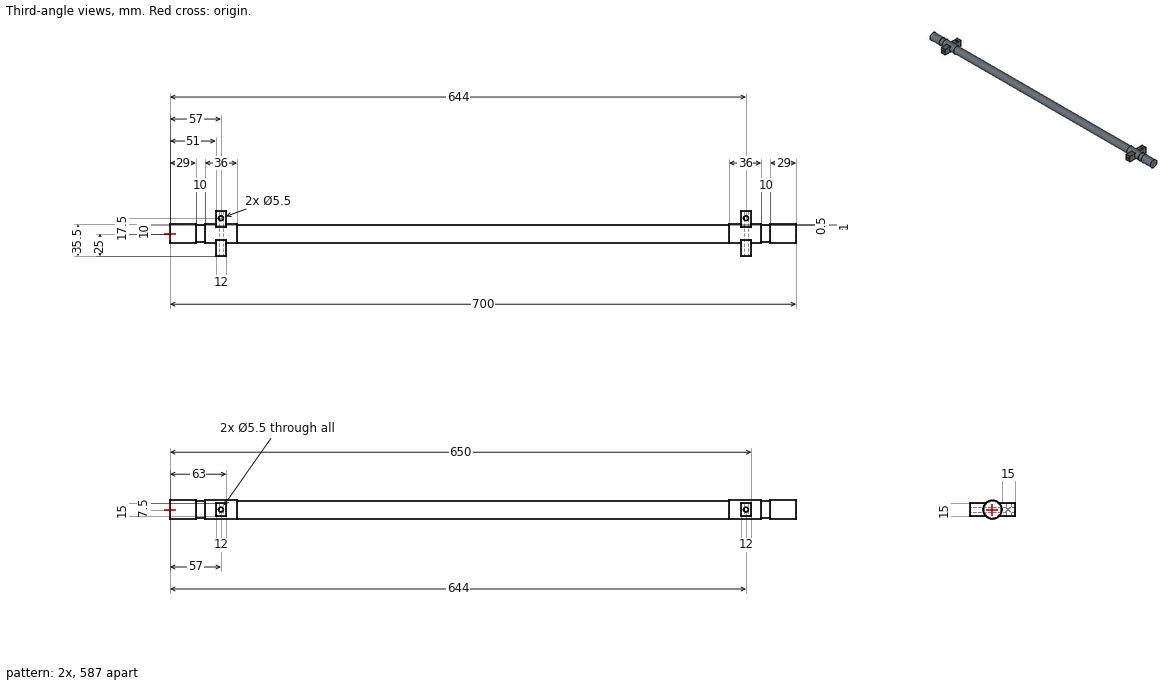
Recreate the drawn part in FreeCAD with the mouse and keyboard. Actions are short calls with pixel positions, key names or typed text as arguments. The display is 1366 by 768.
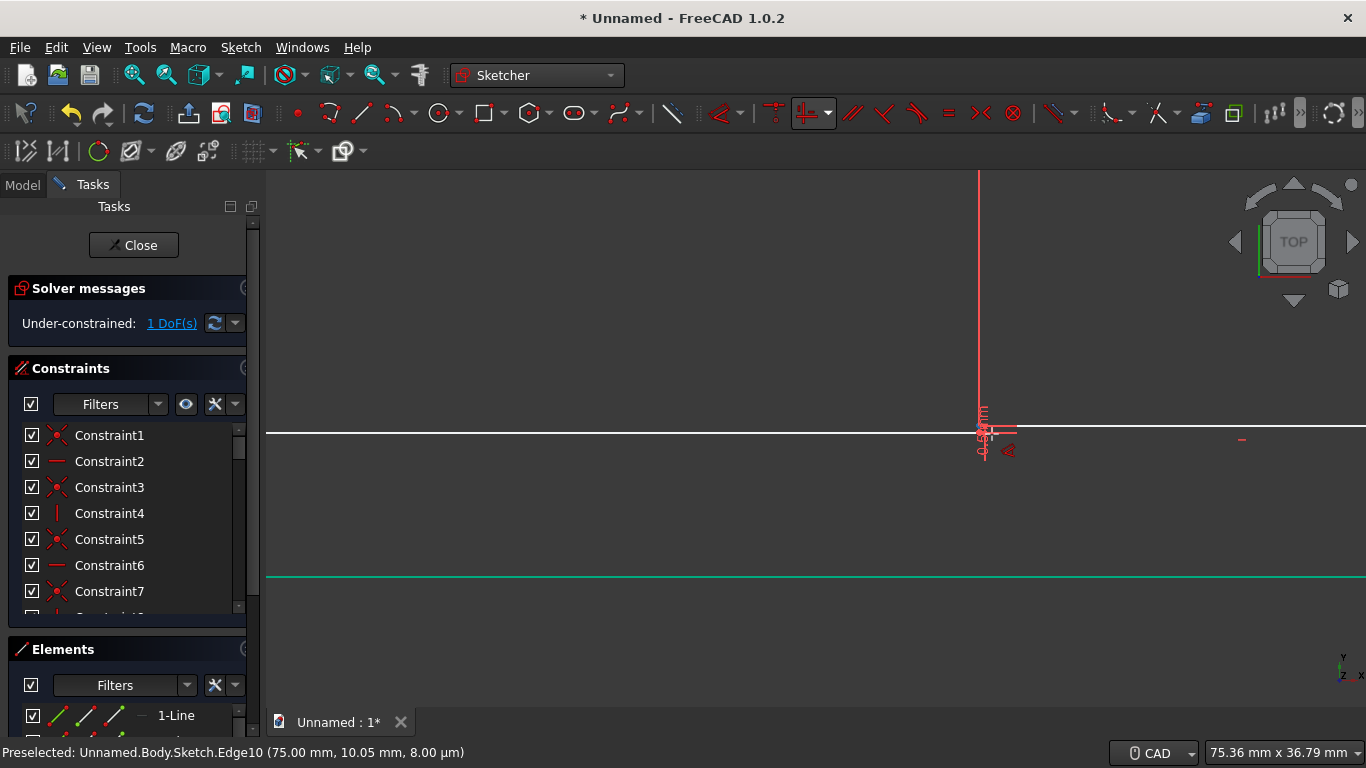
click(979, 433)
click(1013, 505)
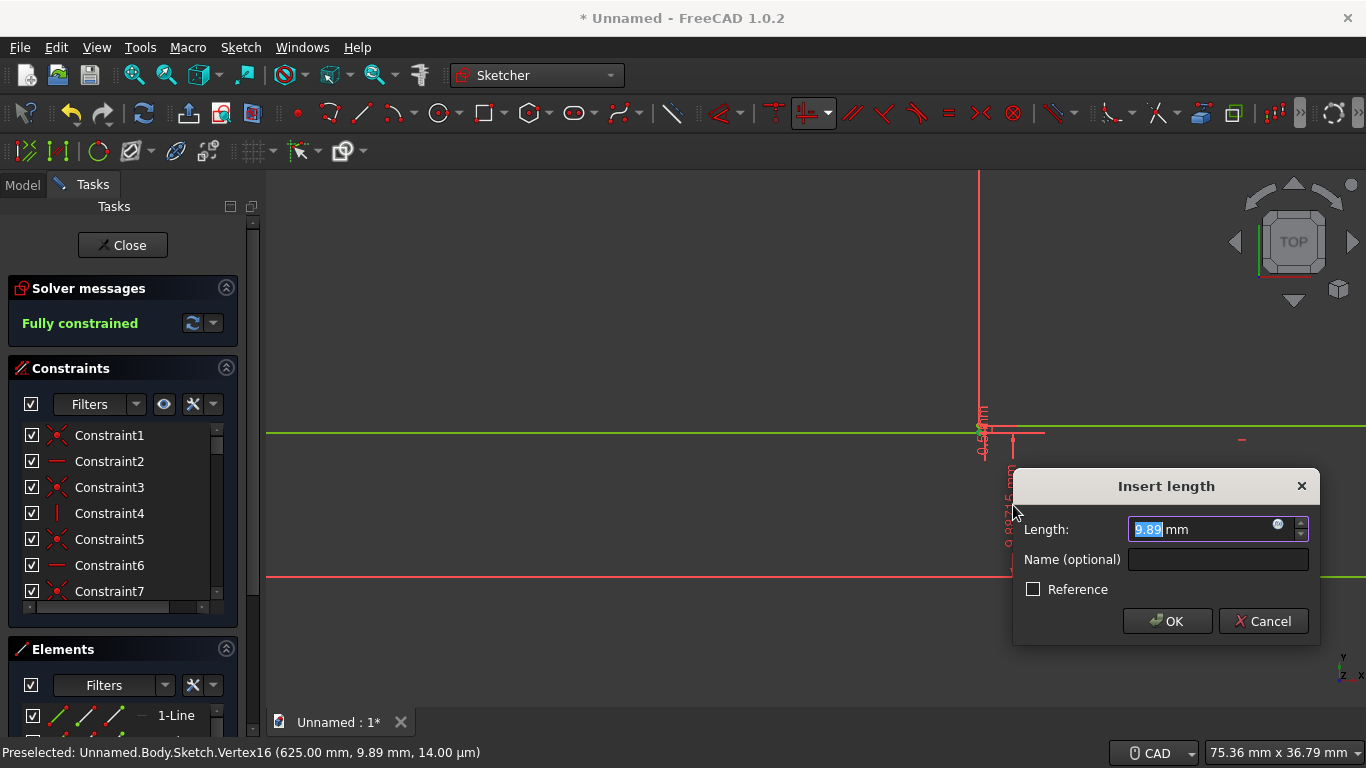
text(10)
key(Return)
key(Escape)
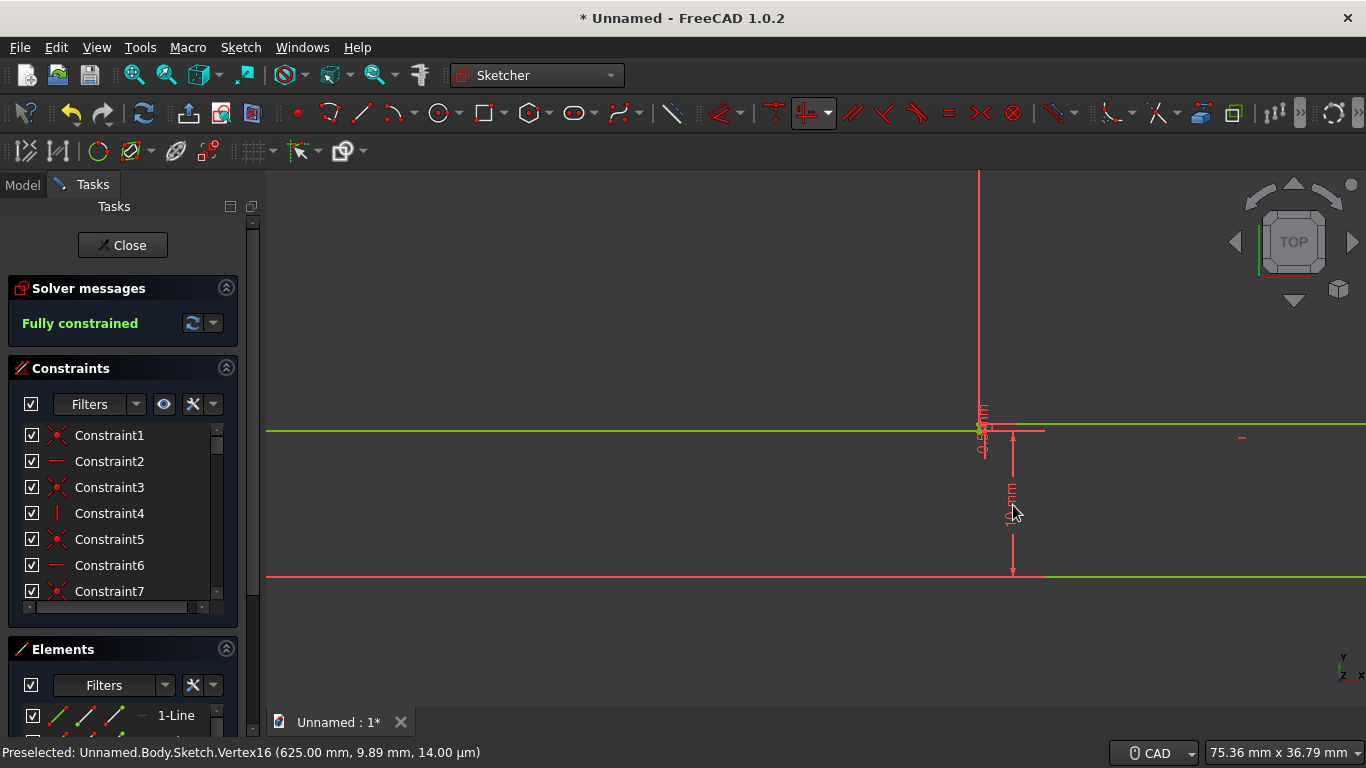
click(123, 245)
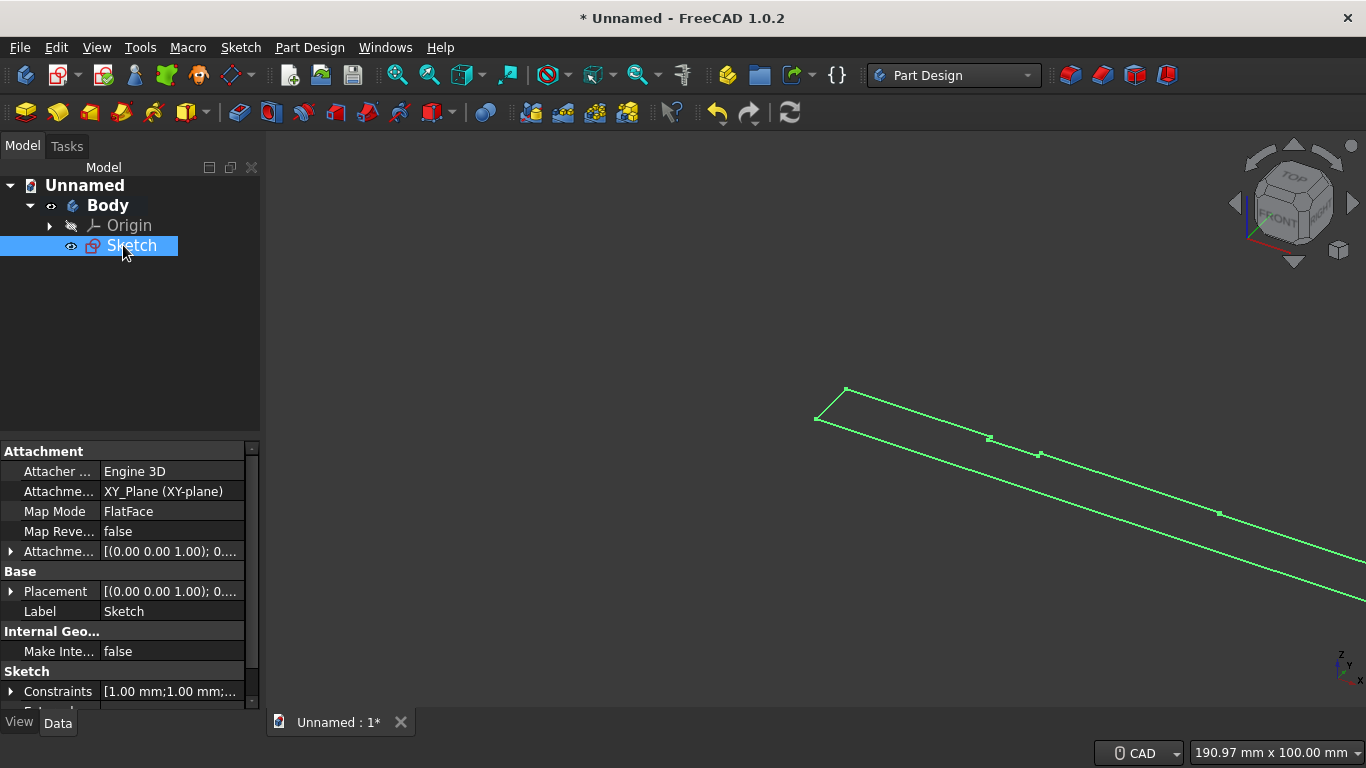
click(58, 112)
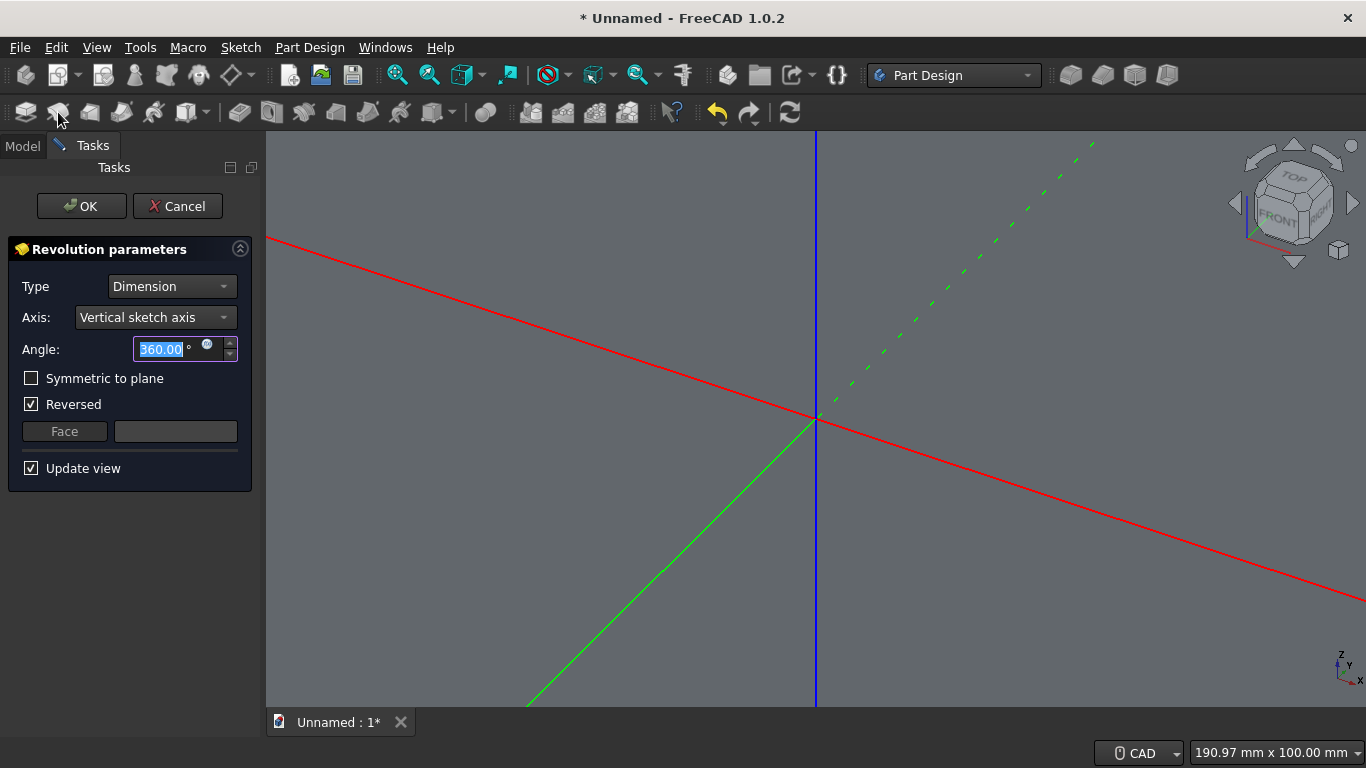
click(156, 318)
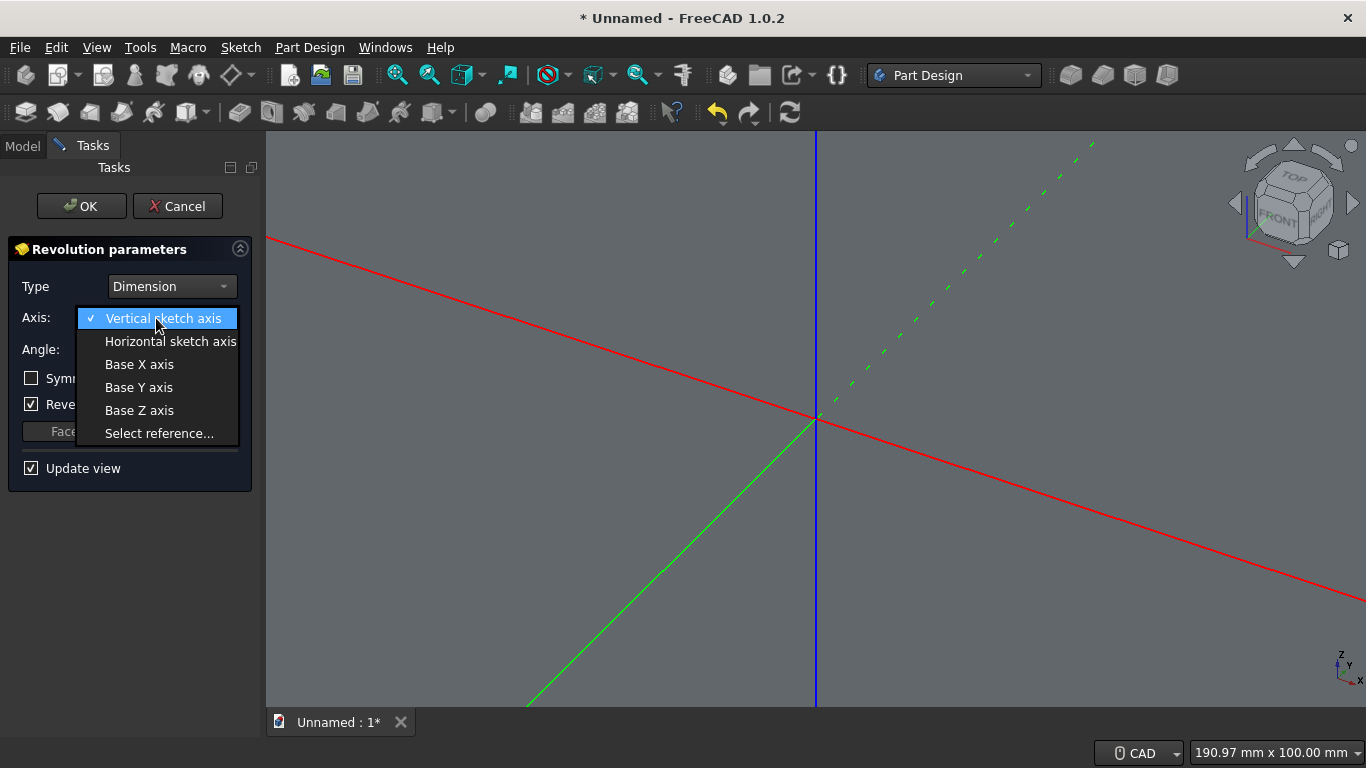
click(156, 342)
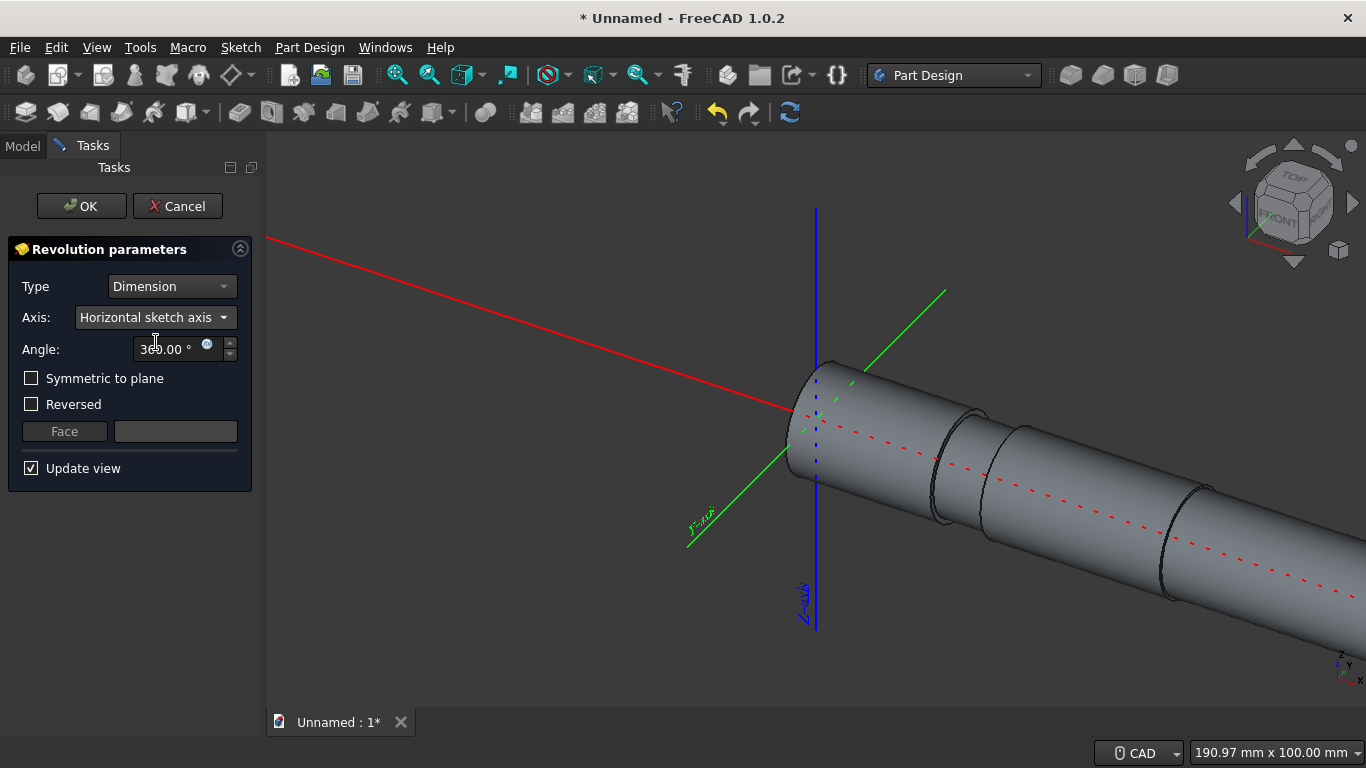
click(82, 206)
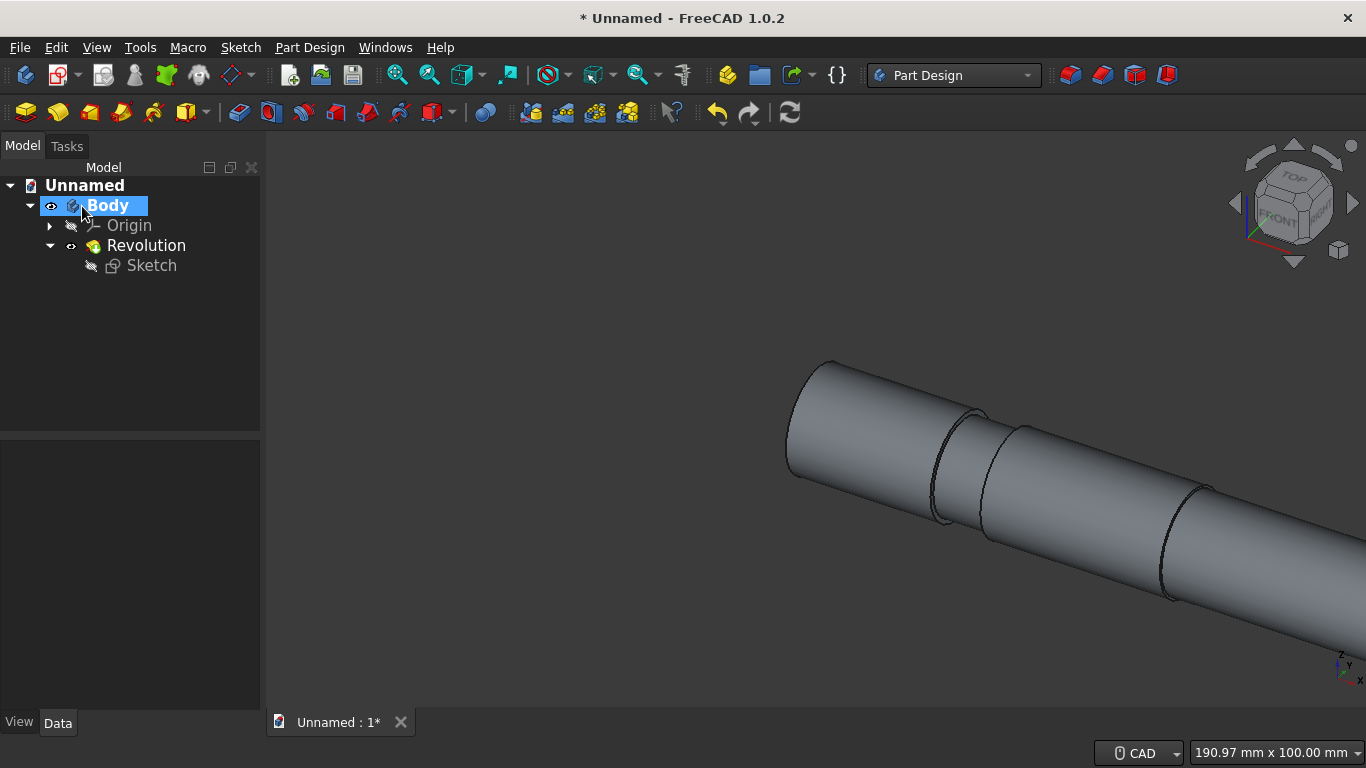
click(398, 76)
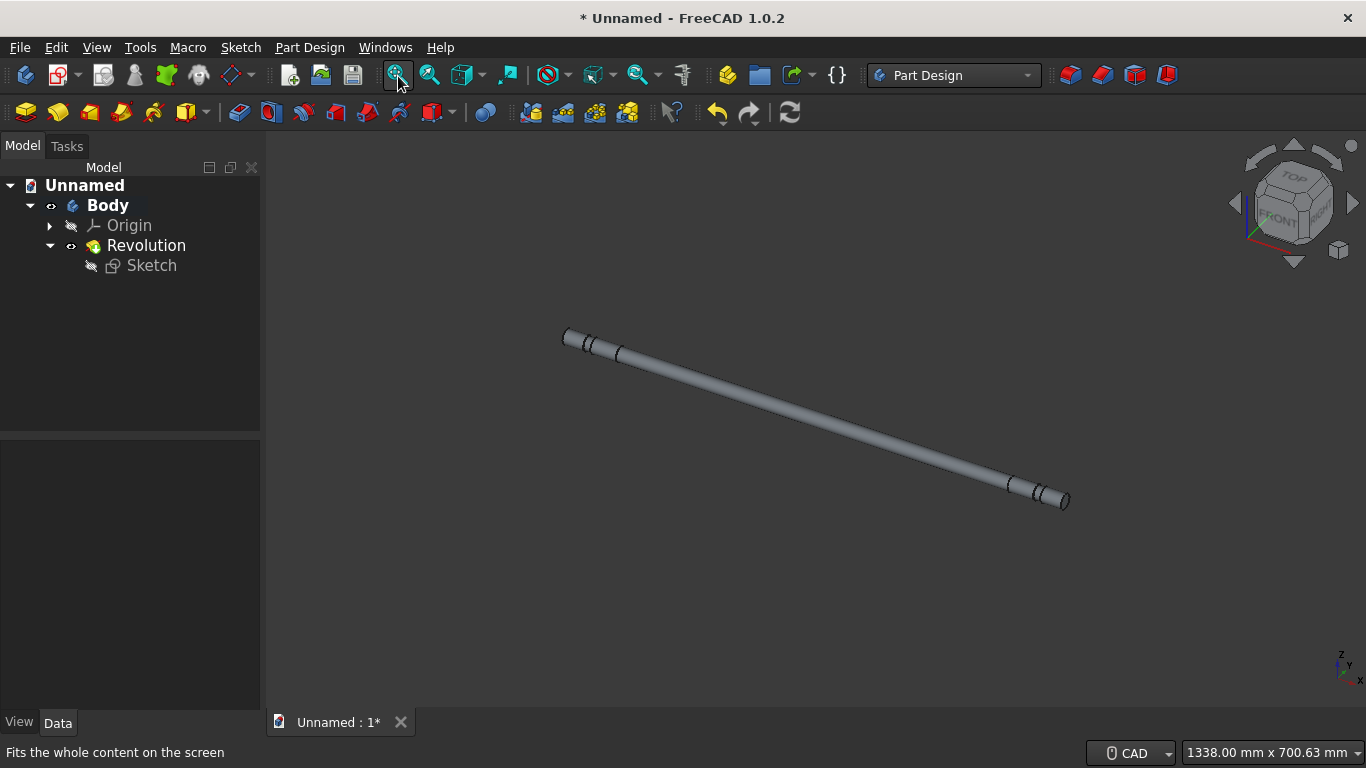
click(58, 76)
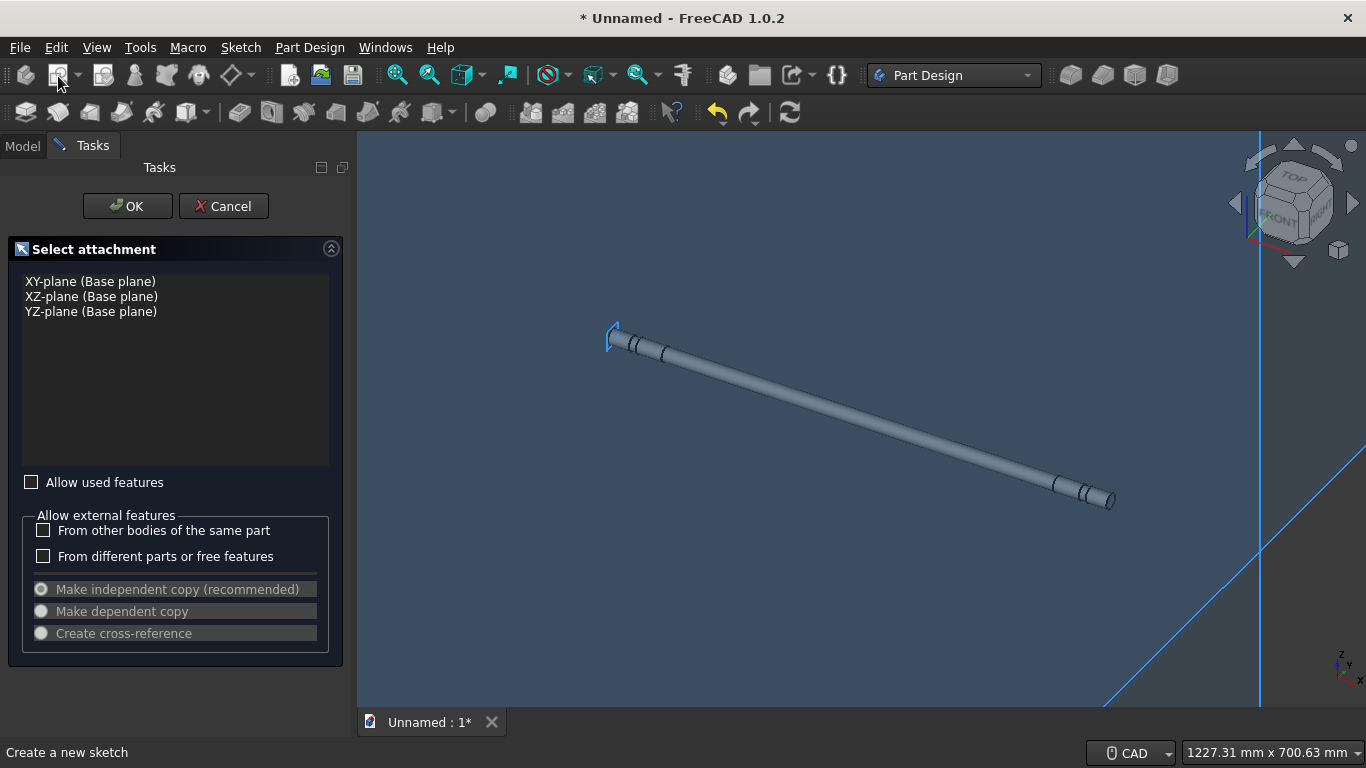
click(82, 282)